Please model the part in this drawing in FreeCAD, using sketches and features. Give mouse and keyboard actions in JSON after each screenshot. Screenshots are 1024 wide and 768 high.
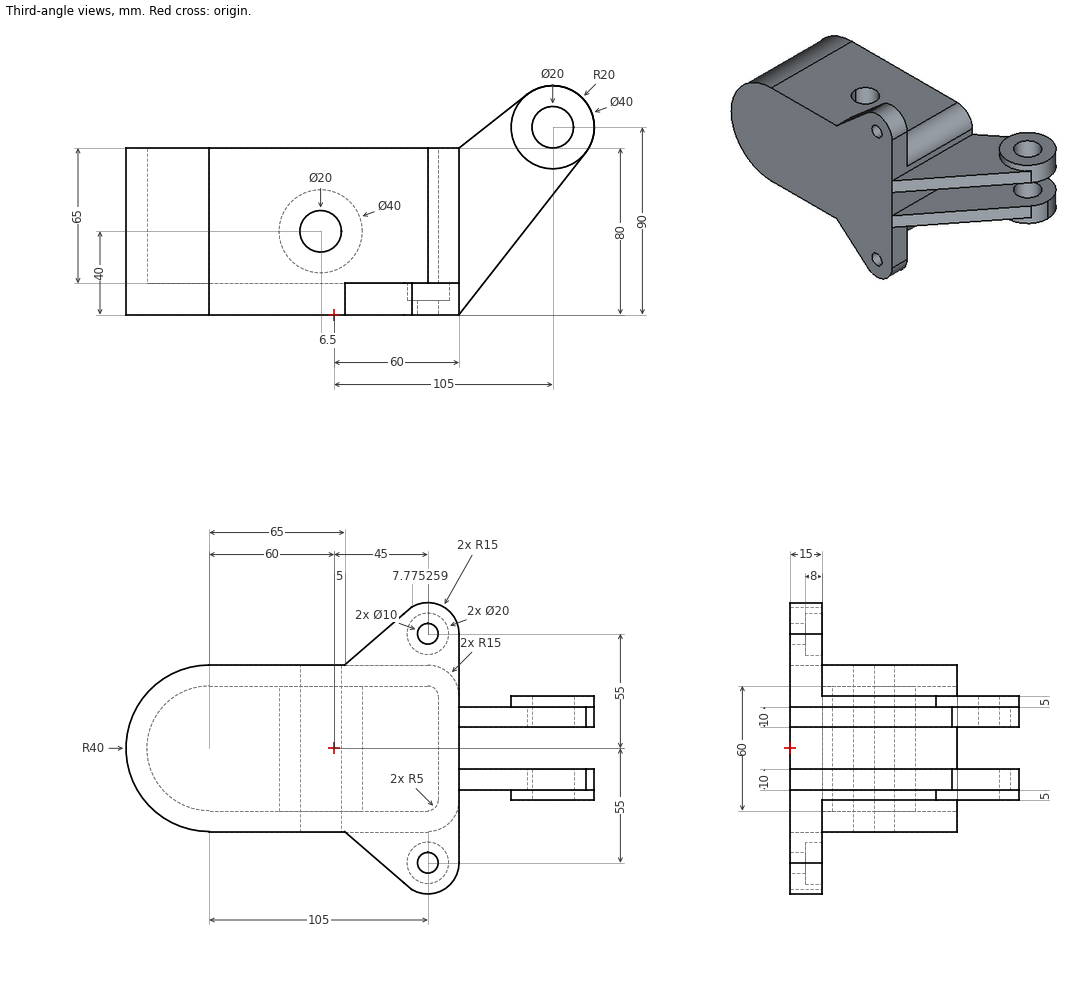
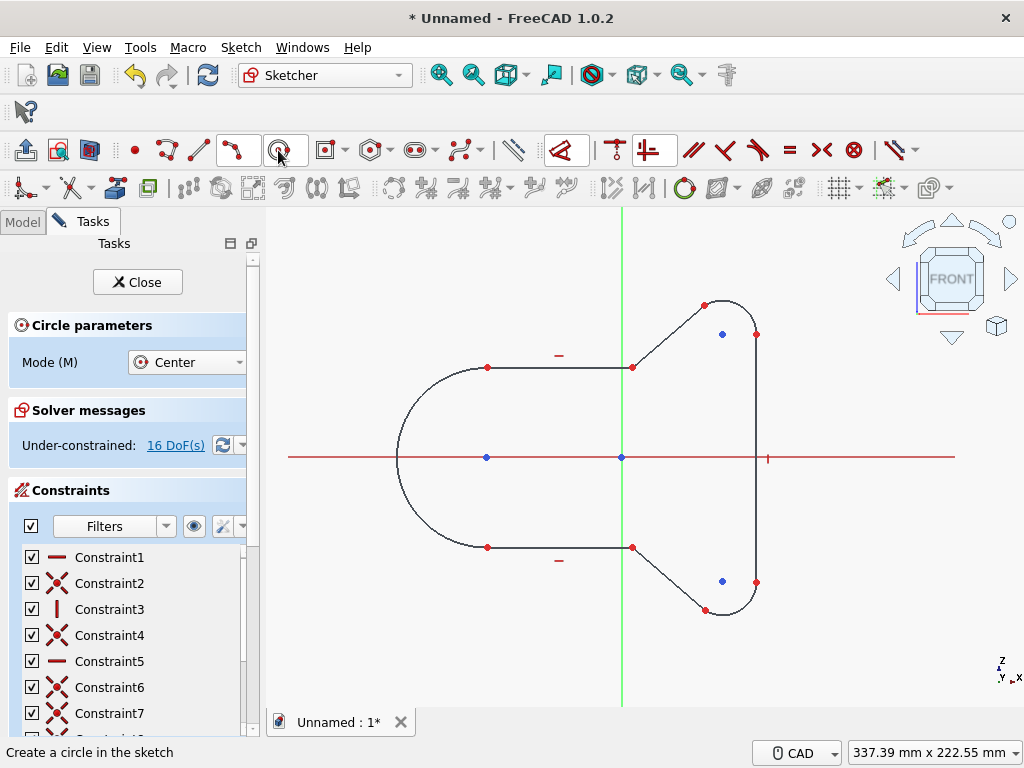
{"action": "scroll", "coordinate": [723, 334], "scroll_direction": "up", "scroll_amount": 4}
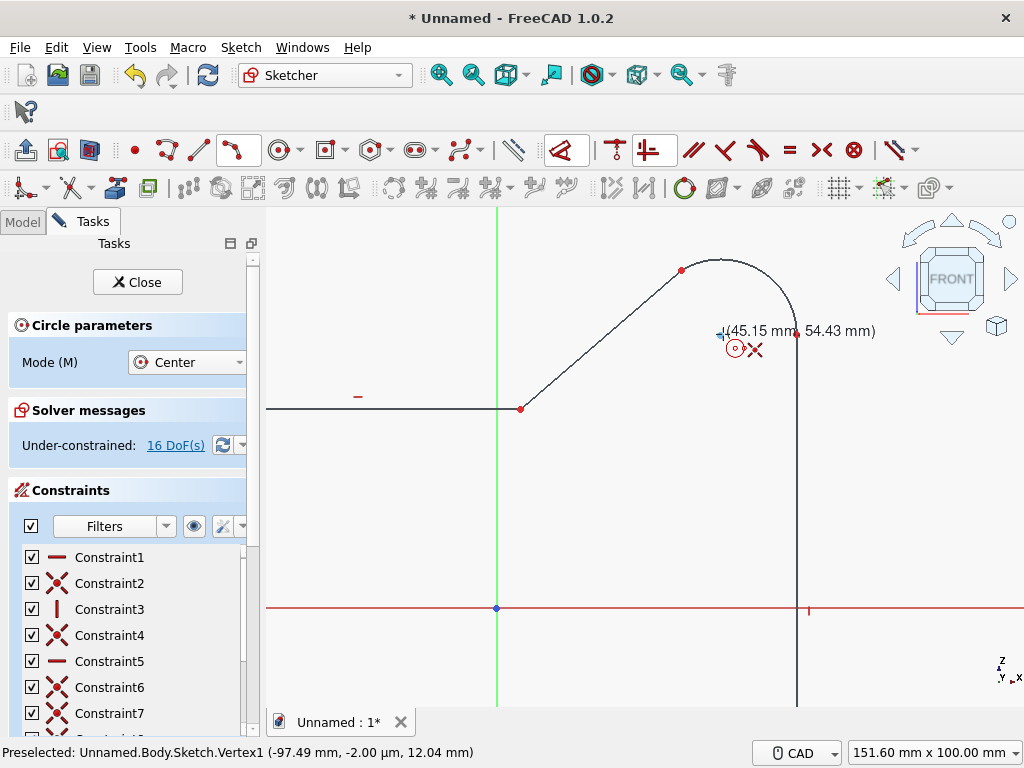
{"action": "left_click", "coordinate": [722, 333]}
{"action": "left_click", "coordinate": [739, 315]}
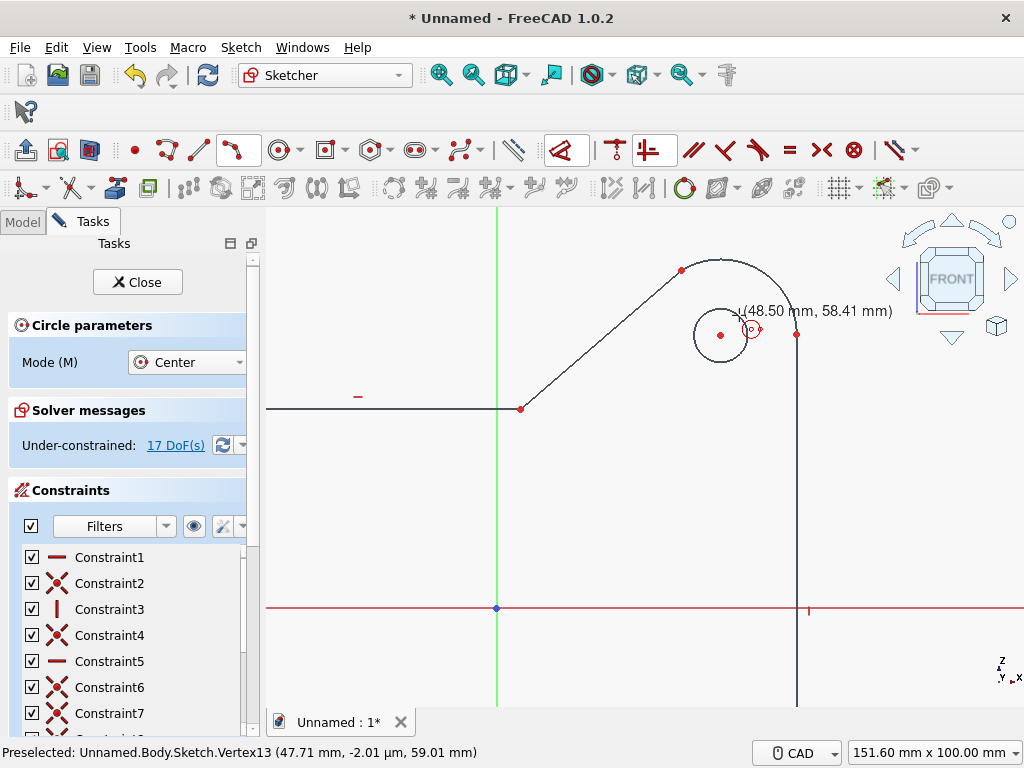
{"action": "scroll", "coordinate": [723, 334], "scroll_direction": "down", "scroll_amount": 4}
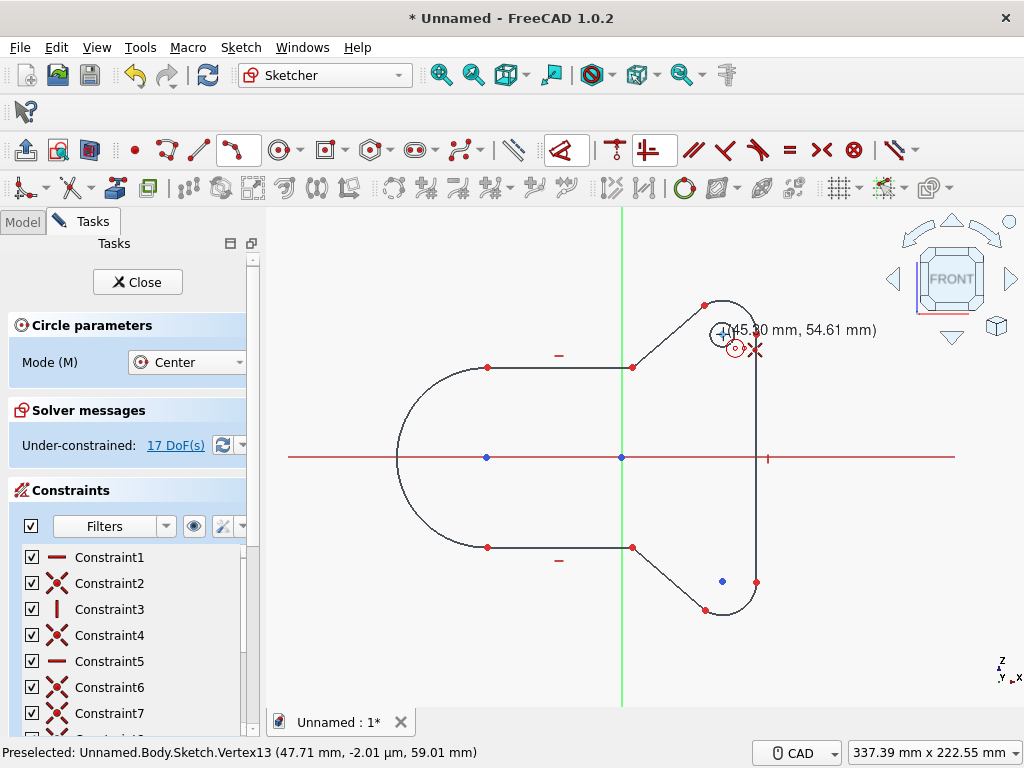
{"action": "scroll", "coordinate": [723, 581], "scroll_direction": "up", "scroll_amount": 4}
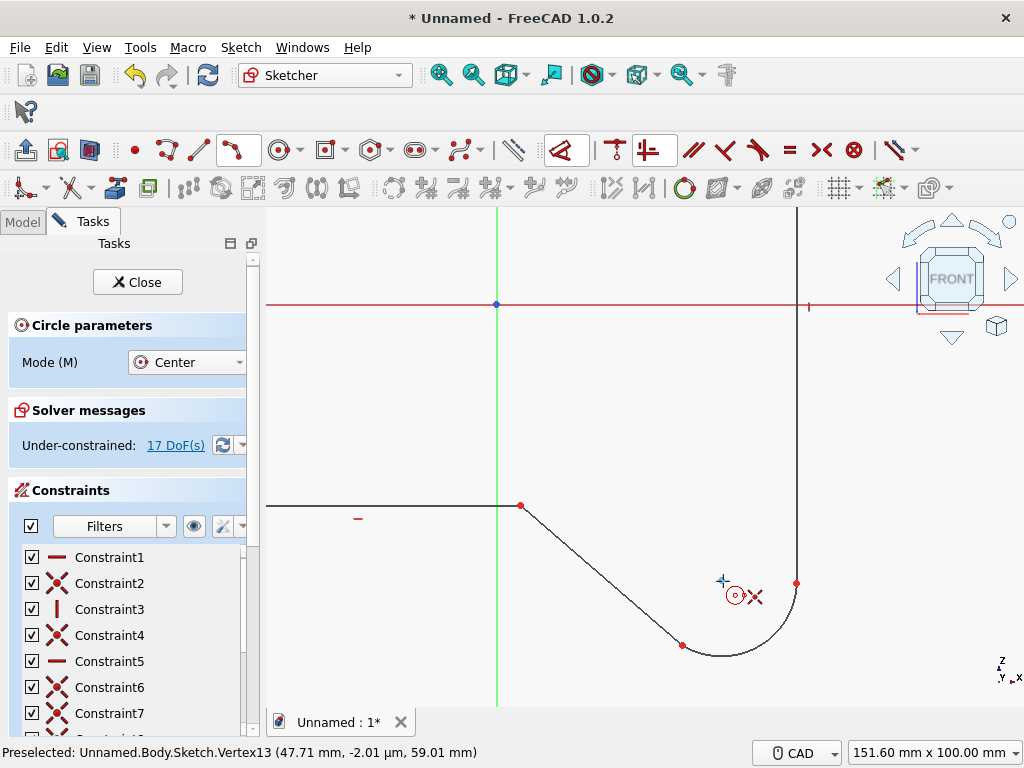
{"action": "left_click", "coordinate": [722, 580]}
{"action": "left_click", "coordinate": [739, 562]}
{"action": "key", "text": "Escape"}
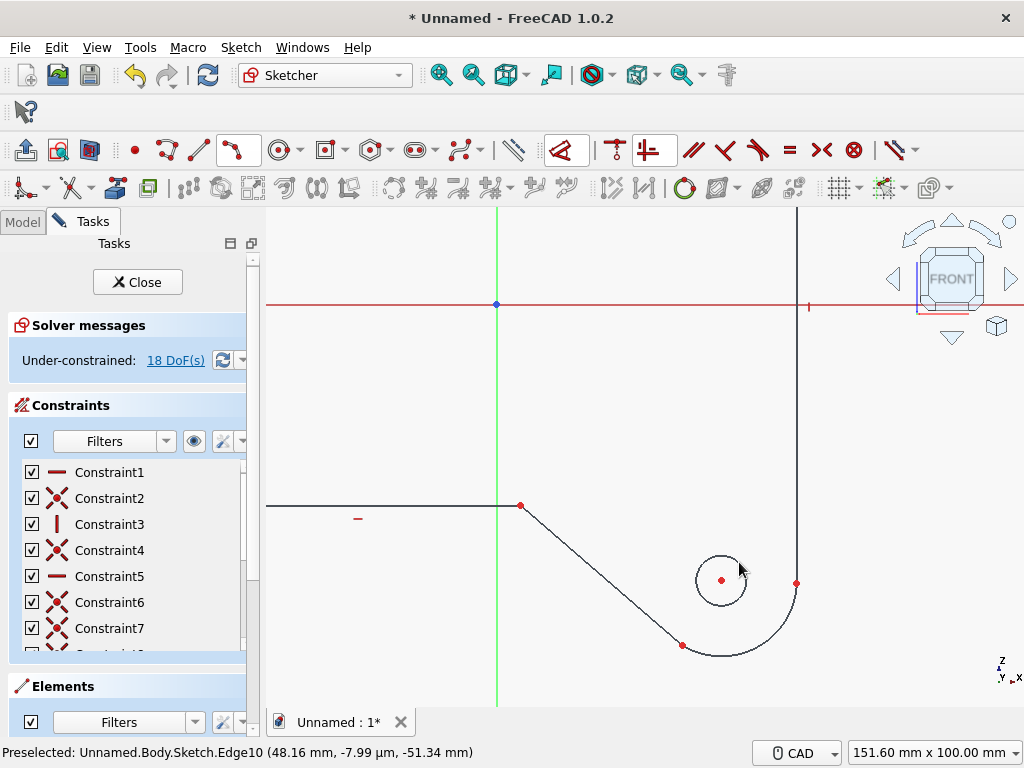
{"action": "left_click", "coordinate": [797, 417]}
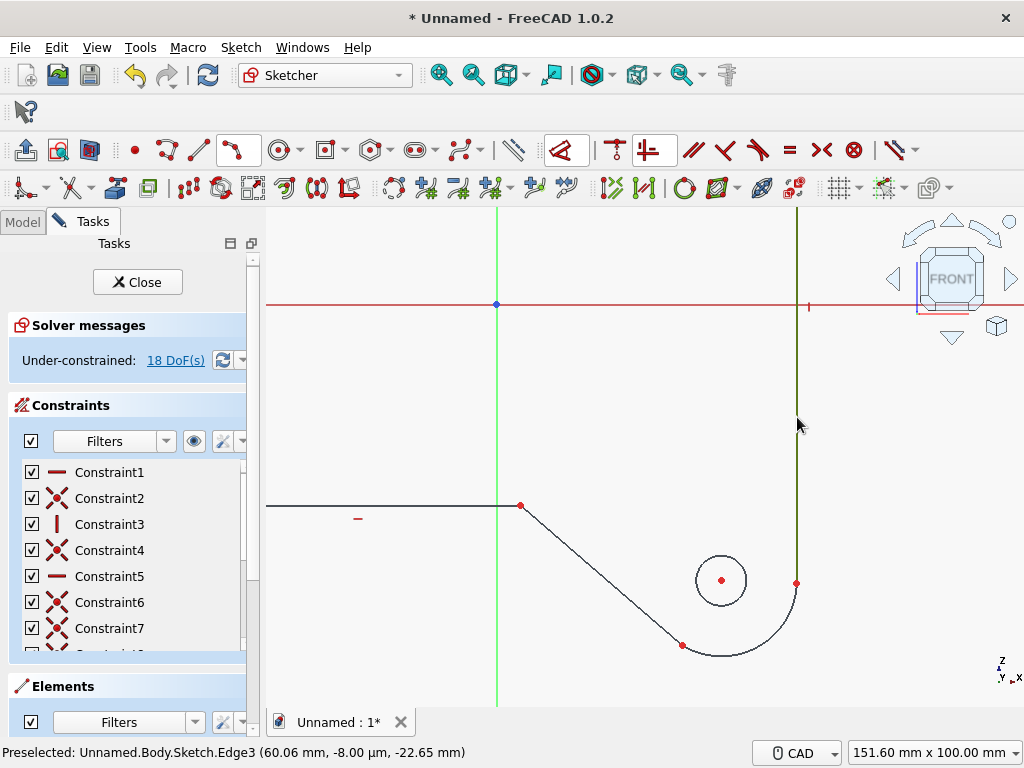
{"action": "scroll", "coordinate": [723, 581], "scroll_direction": "down", "scroll_amount": 4}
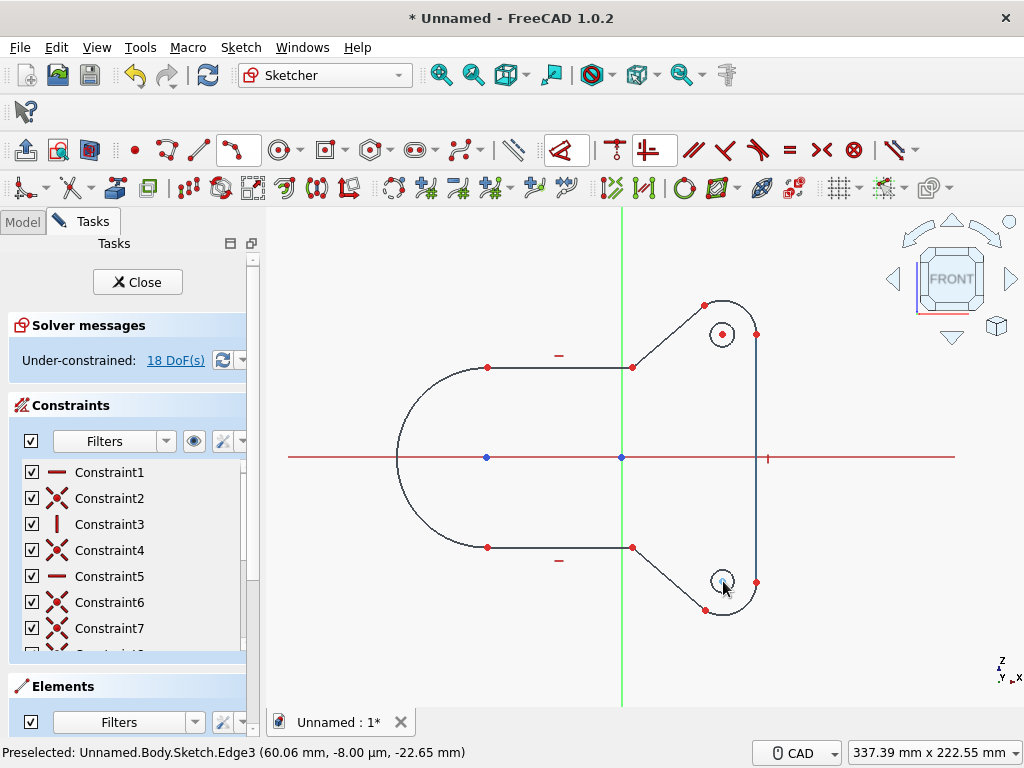
{"action": "left_click", "coordinate": [750, 314]}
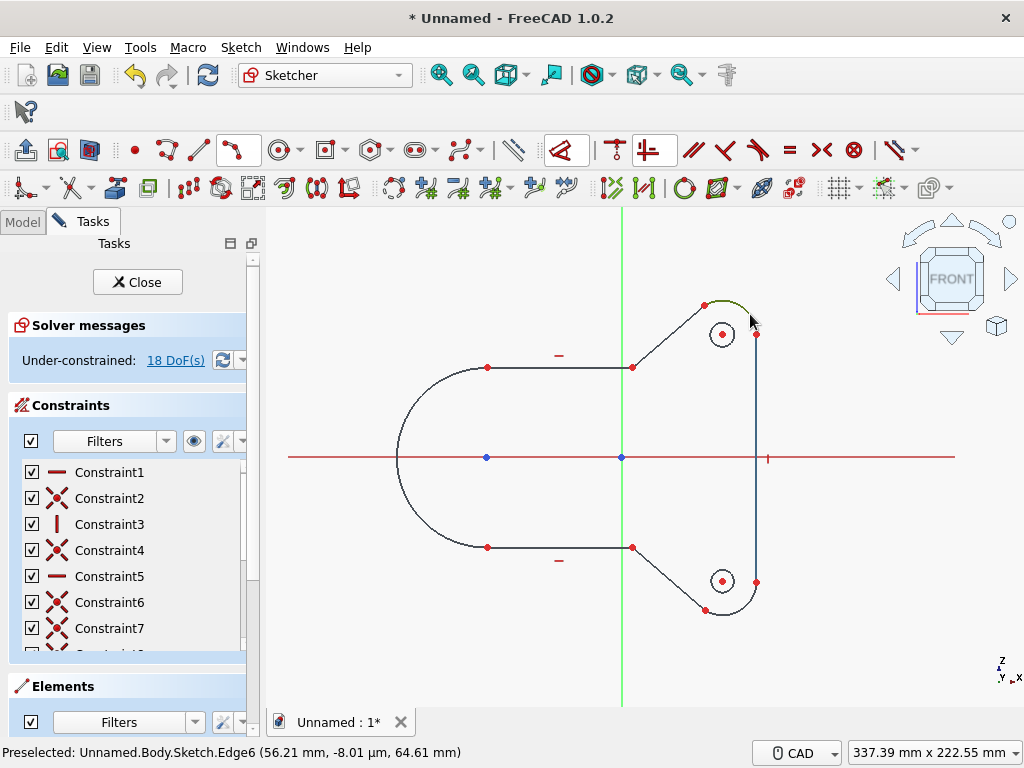
{"action": "left_click", "coordinate": [758, 150]}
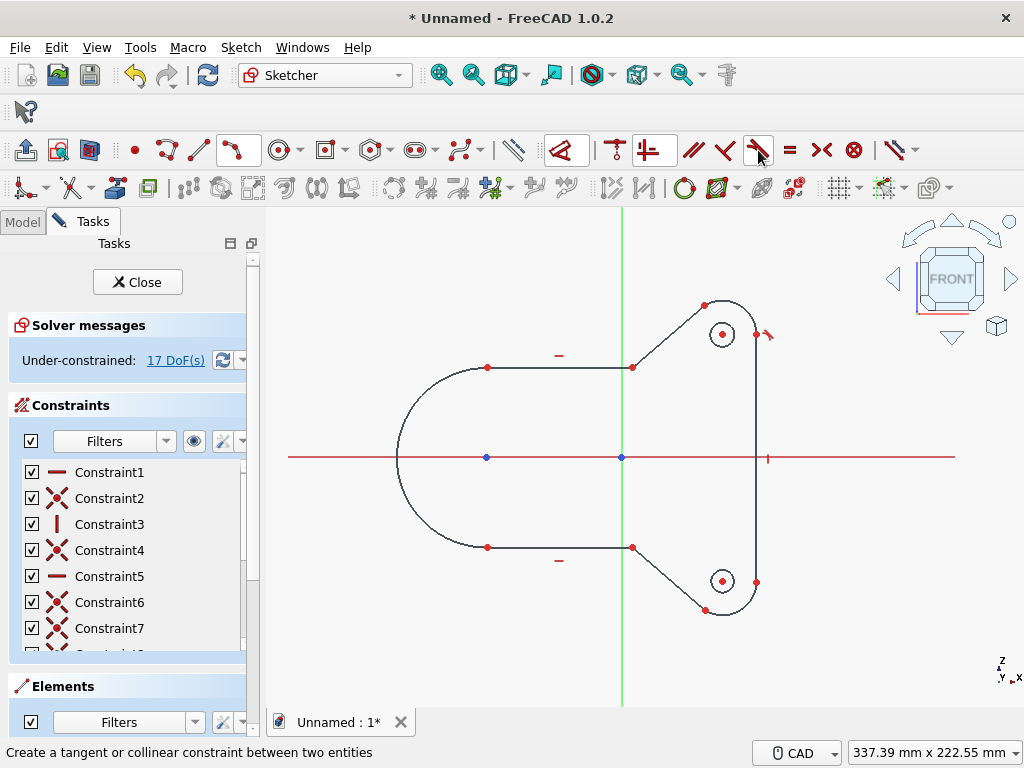
{"action": "left_click", "coordinate": [756, 409]}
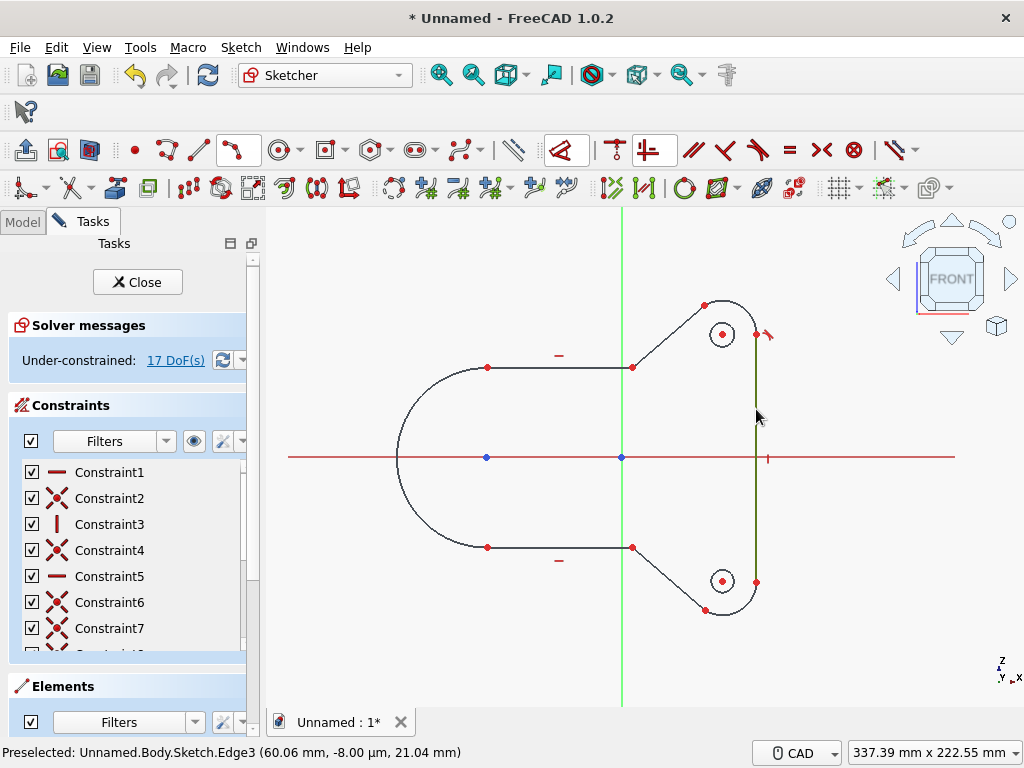
{"action": "left_click", "coordinate": [725, 615]}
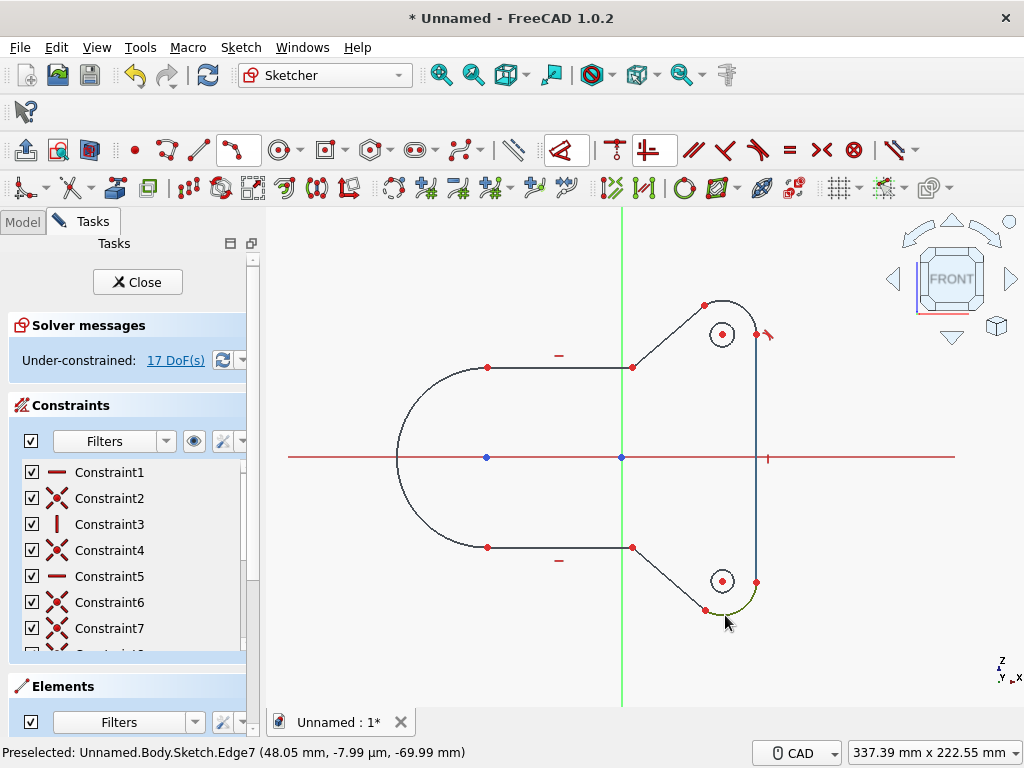
{"action": "left_click", "coordinate": [758, 150]}